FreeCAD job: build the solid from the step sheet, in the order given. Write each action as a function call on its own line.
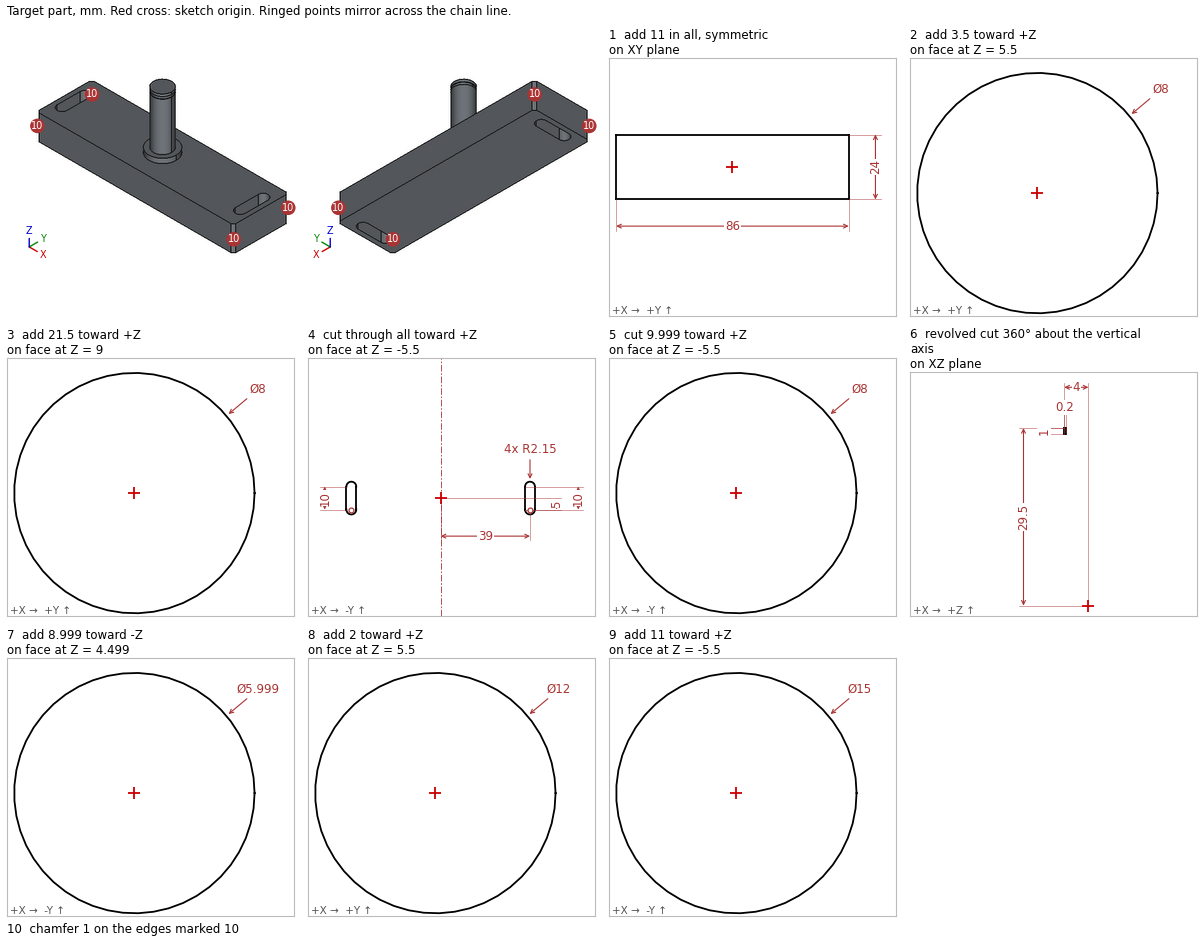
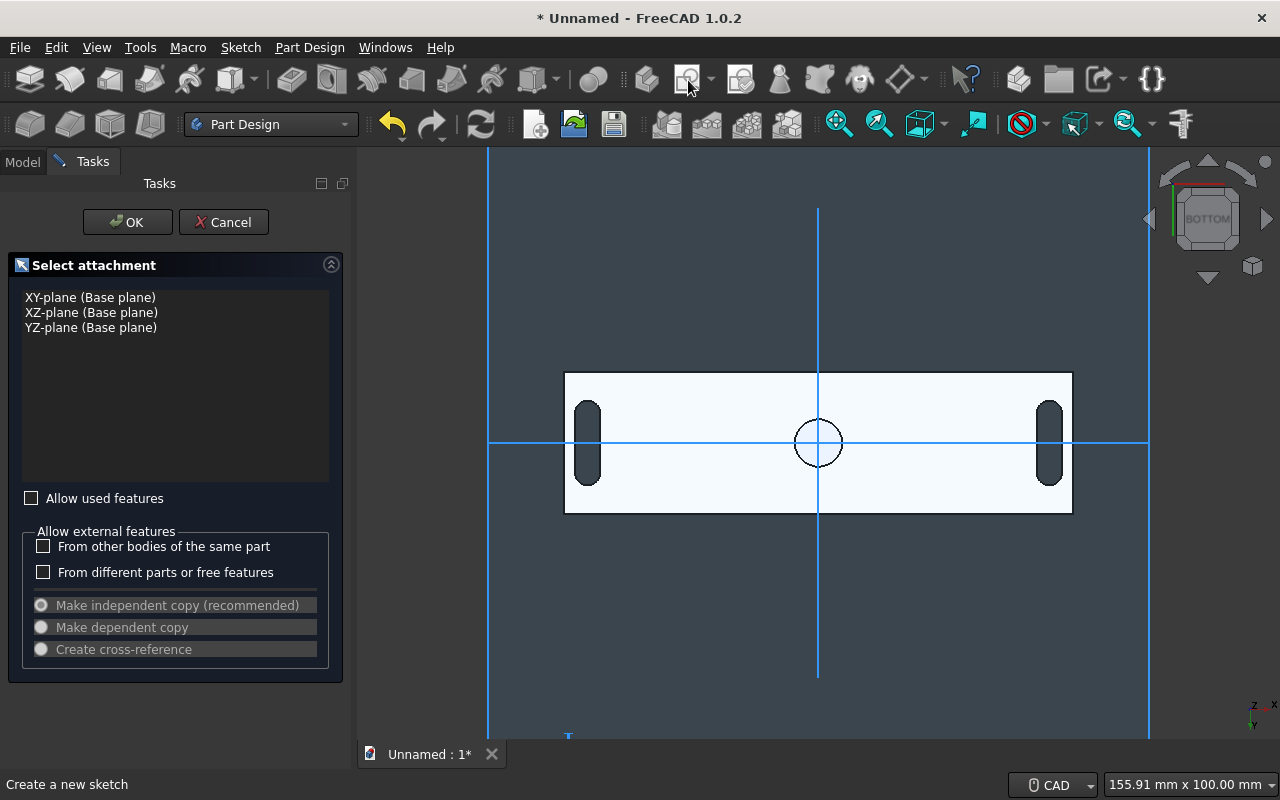
click(82, 312)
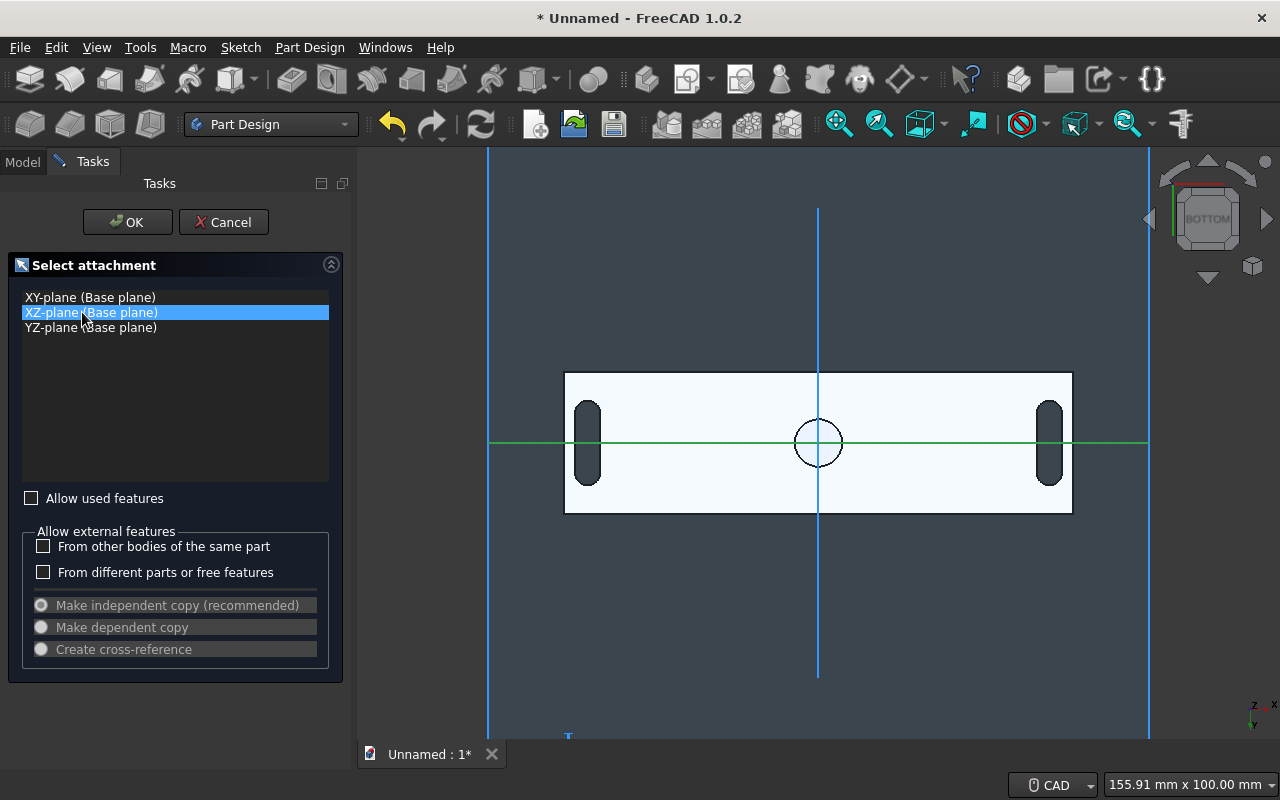
click(128, 222)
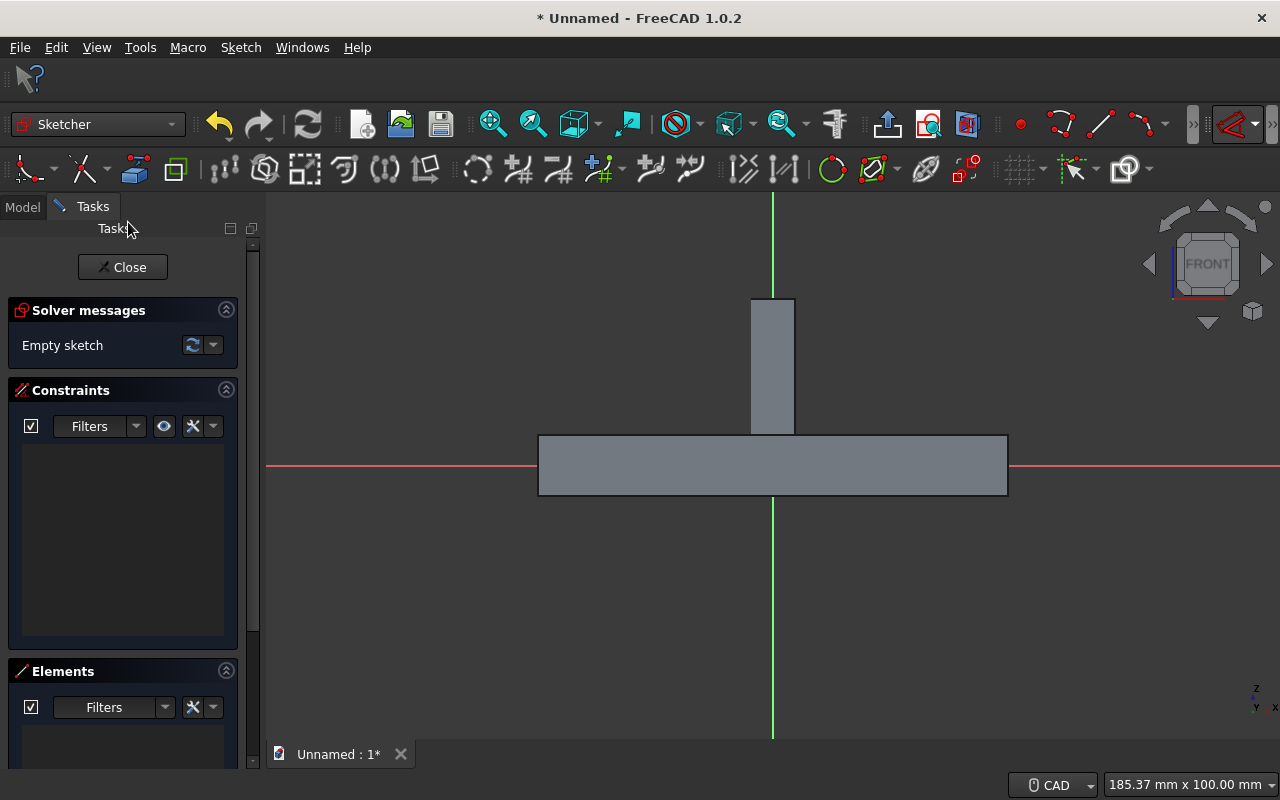
click(968, 124)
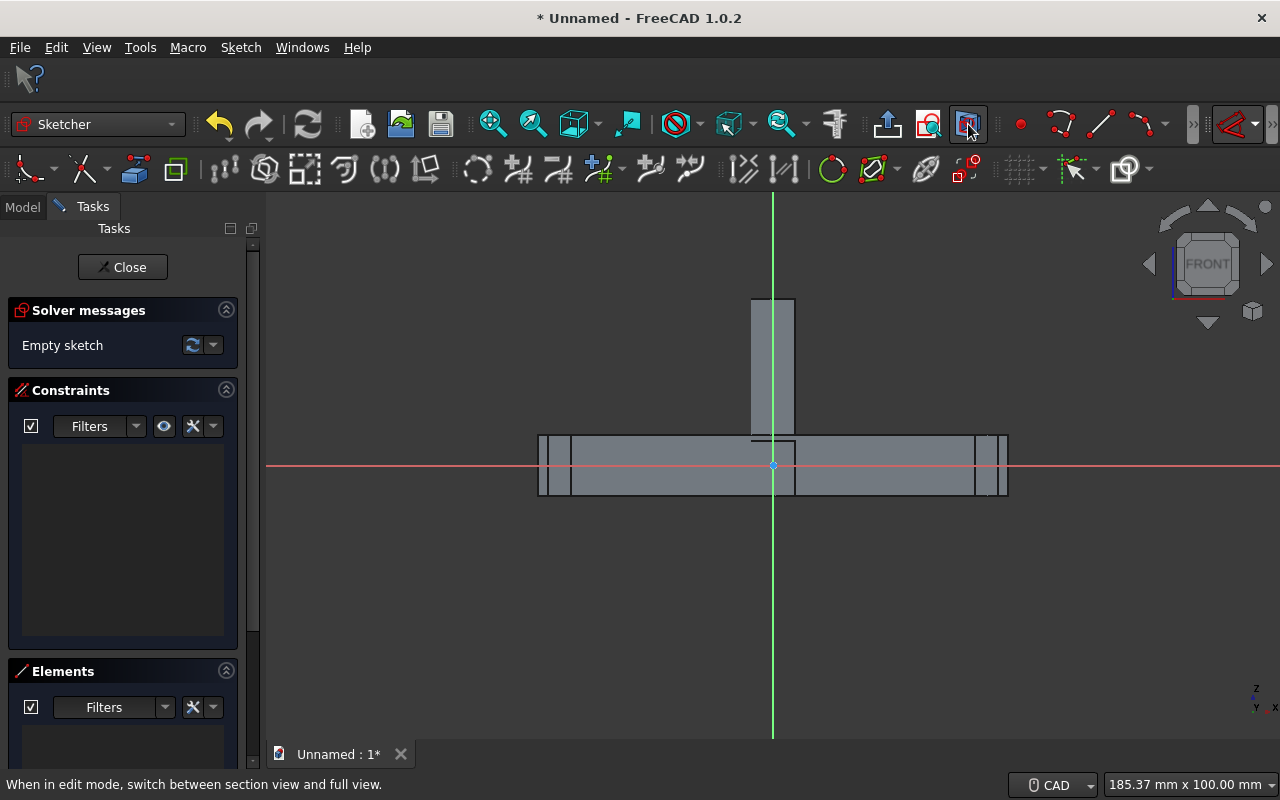
scroll(754, 299, up, 15)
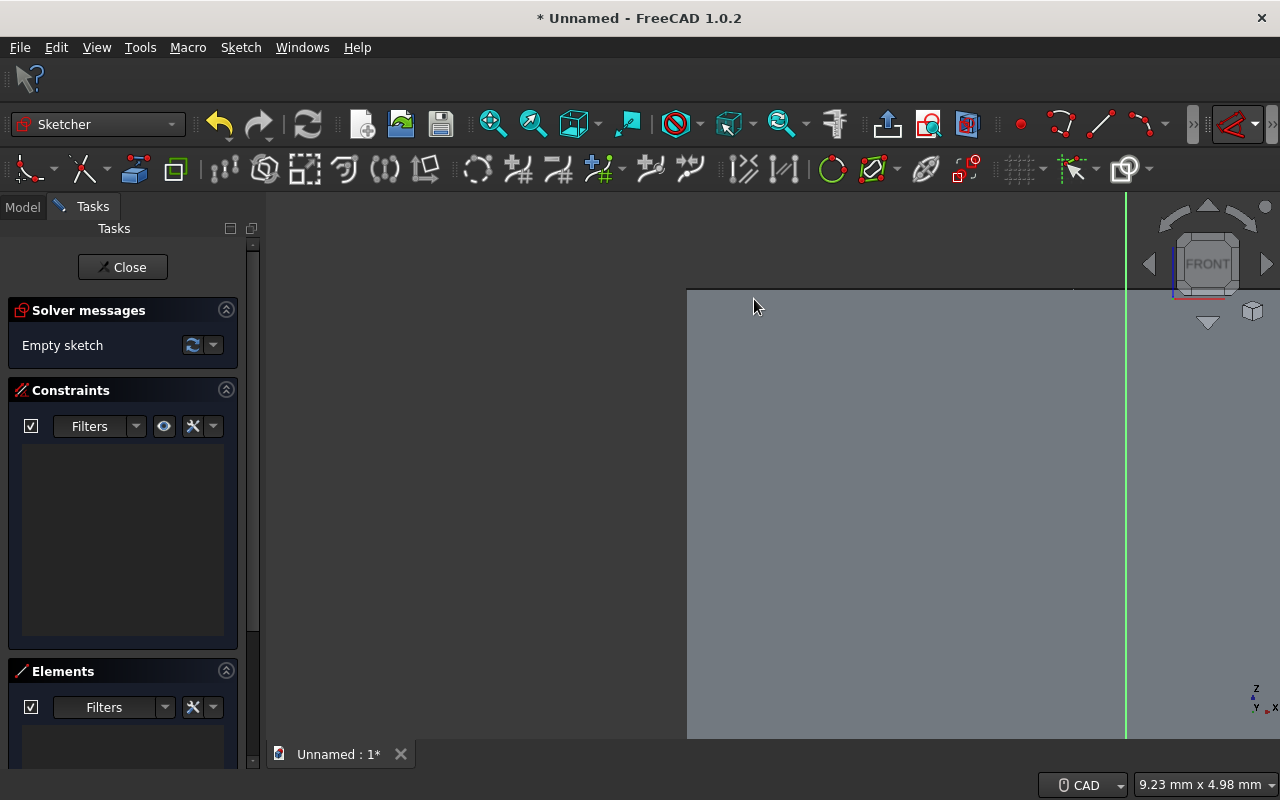
scroll(695, 448, up, 6)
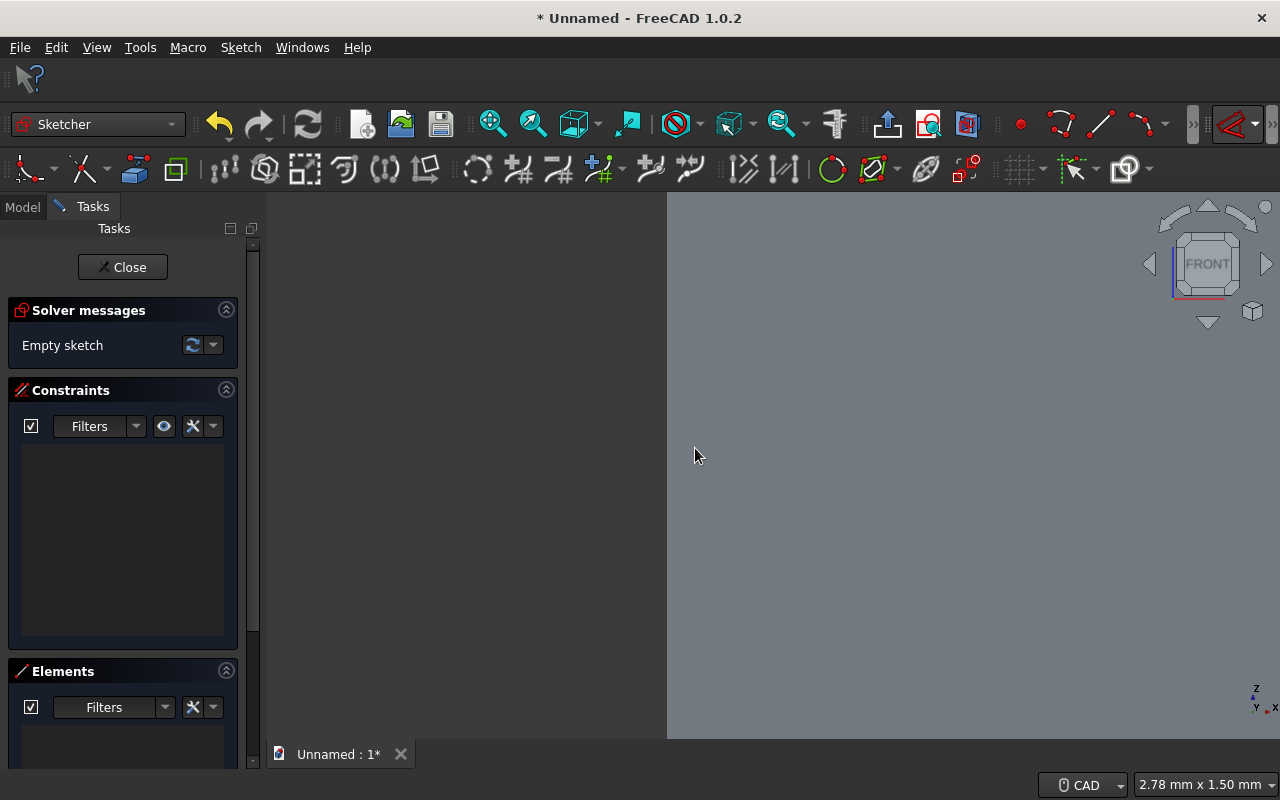
key(g)
key(r)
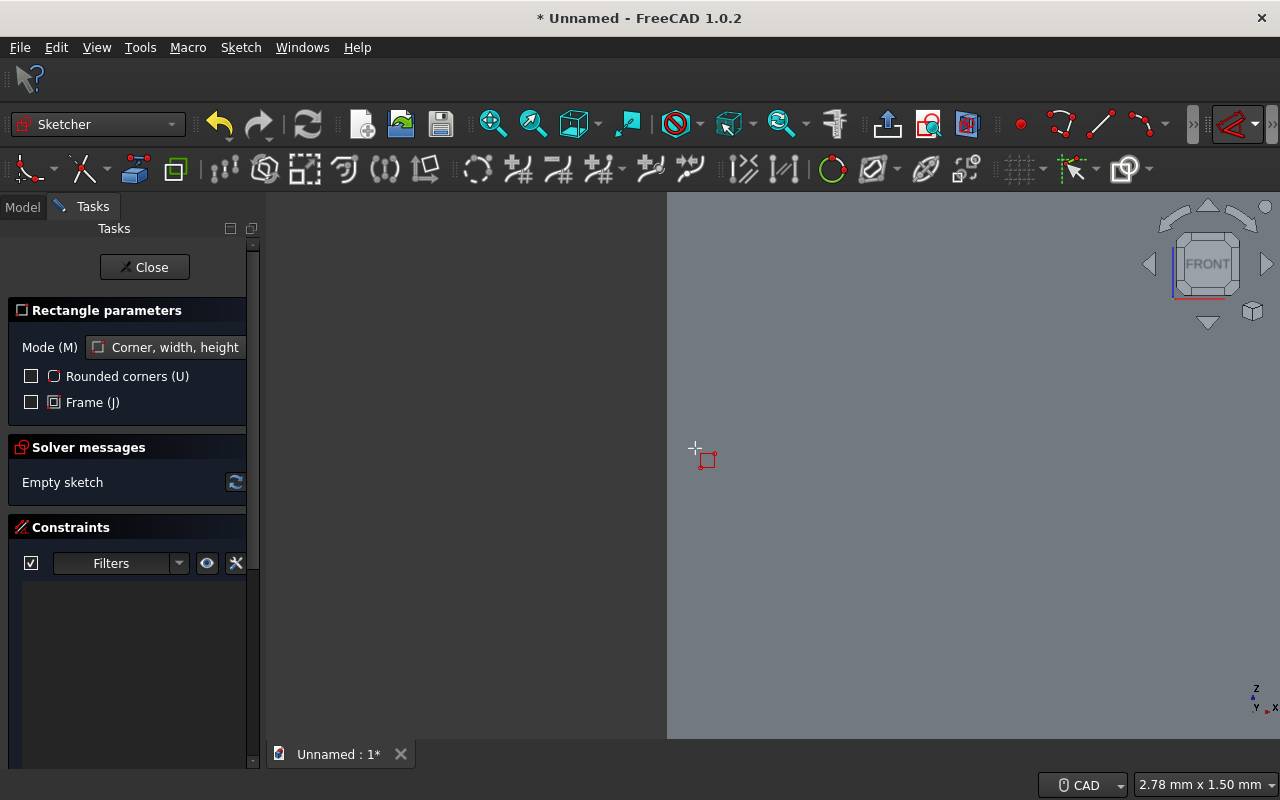
click(667, 282)
click(740, 647)
key(Escape)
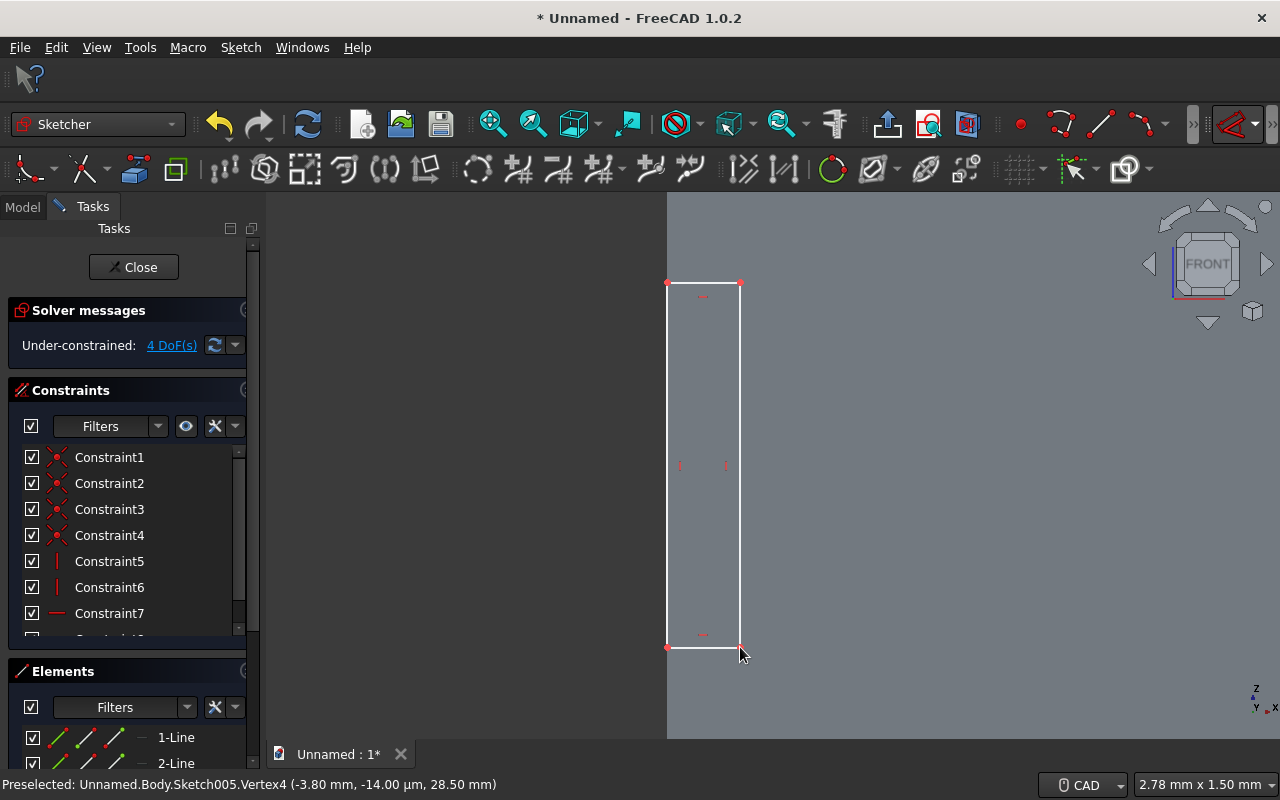
click(667, 393)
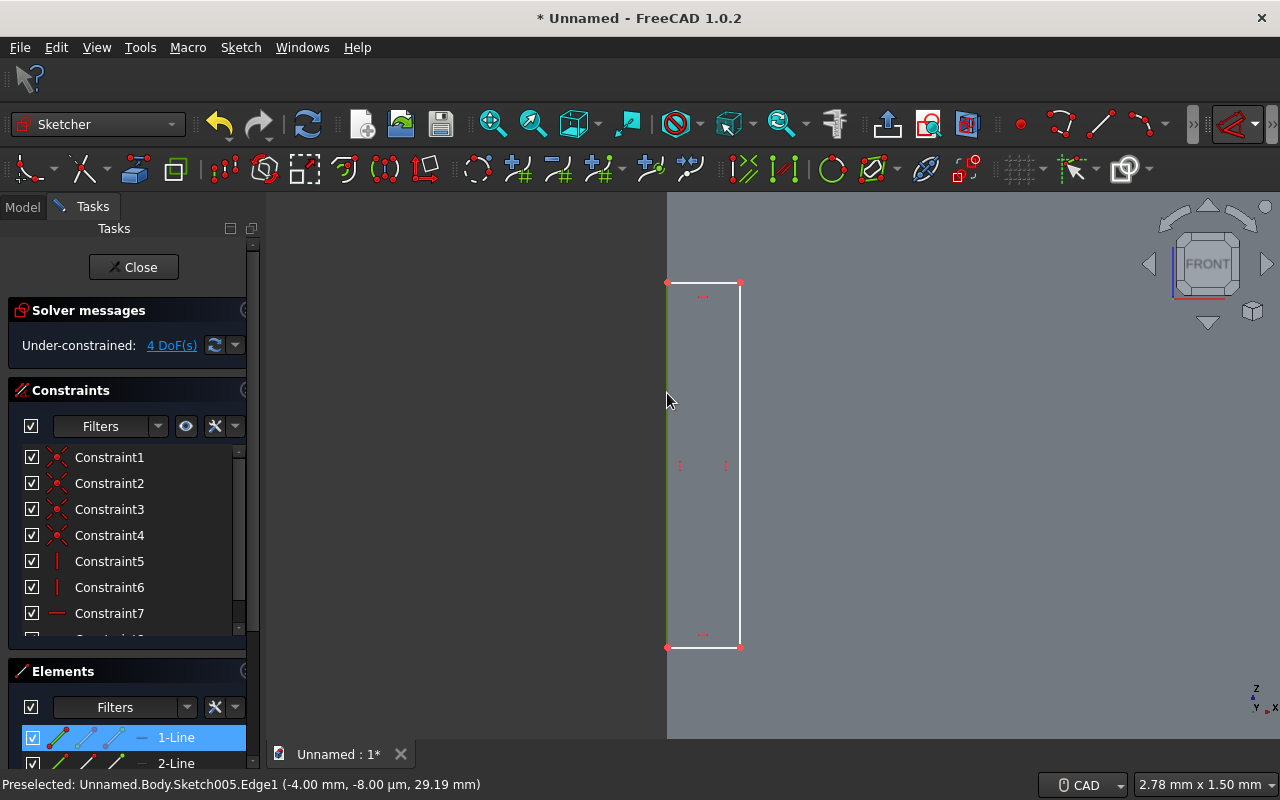
click(1258, 124)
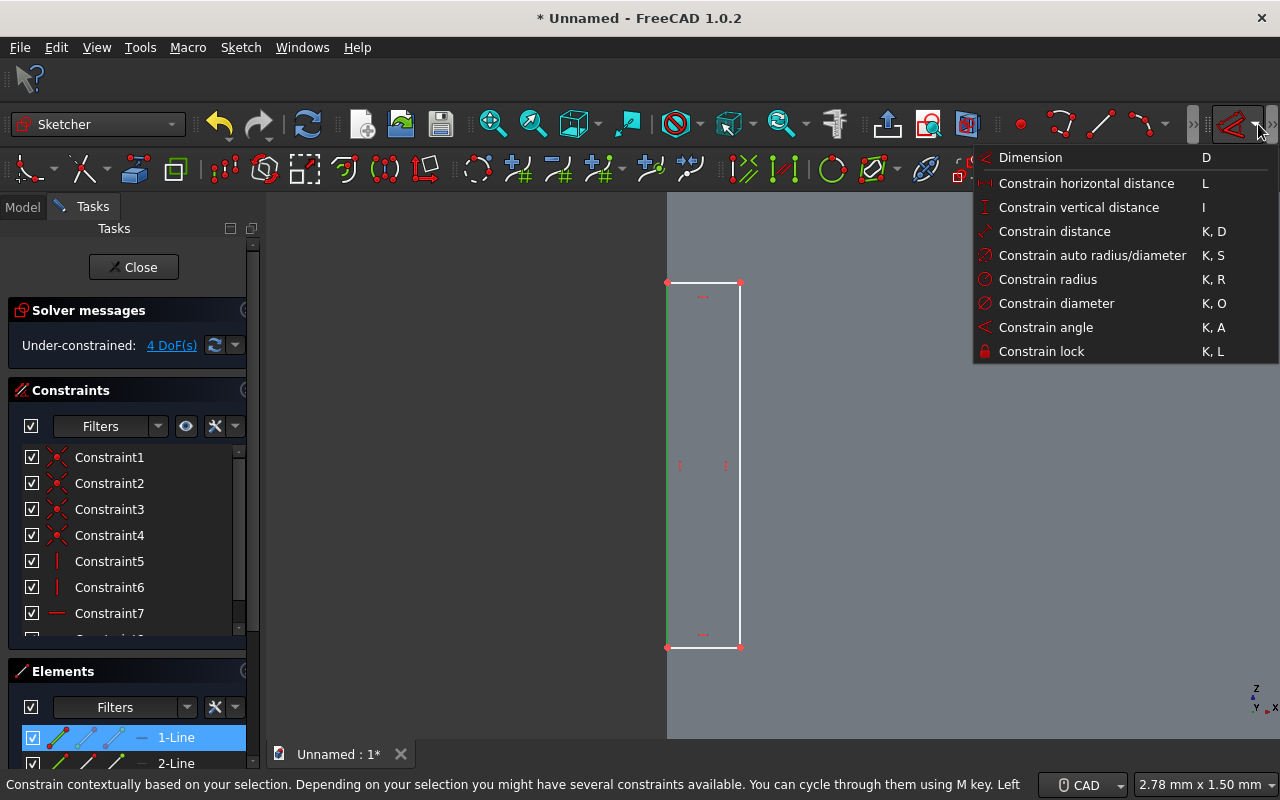
click(1126, 207)